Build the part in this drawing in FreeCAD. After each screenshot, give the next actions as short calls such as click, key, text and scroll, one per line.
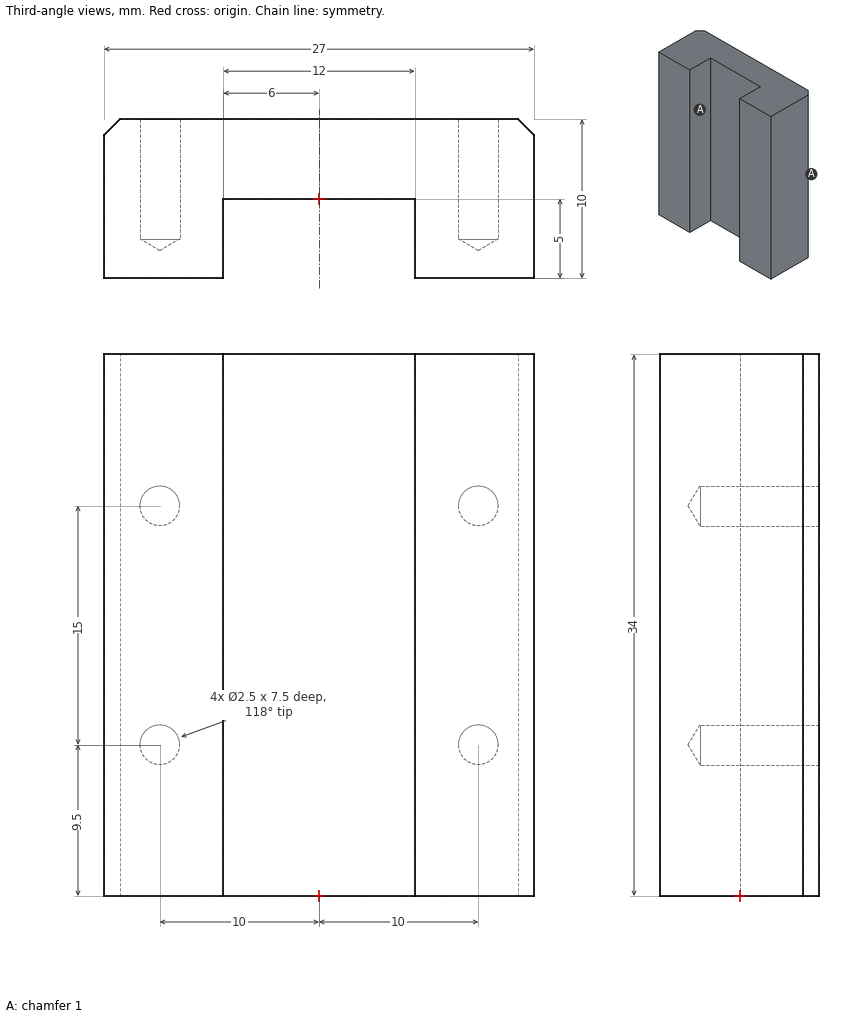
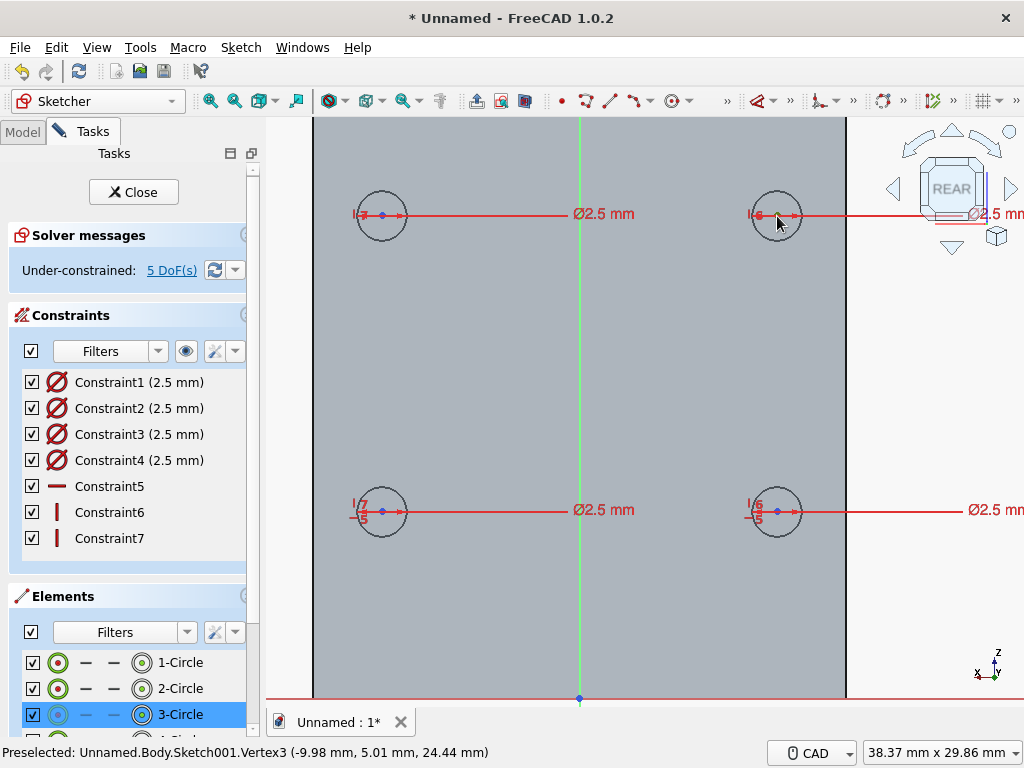
click(382, 216)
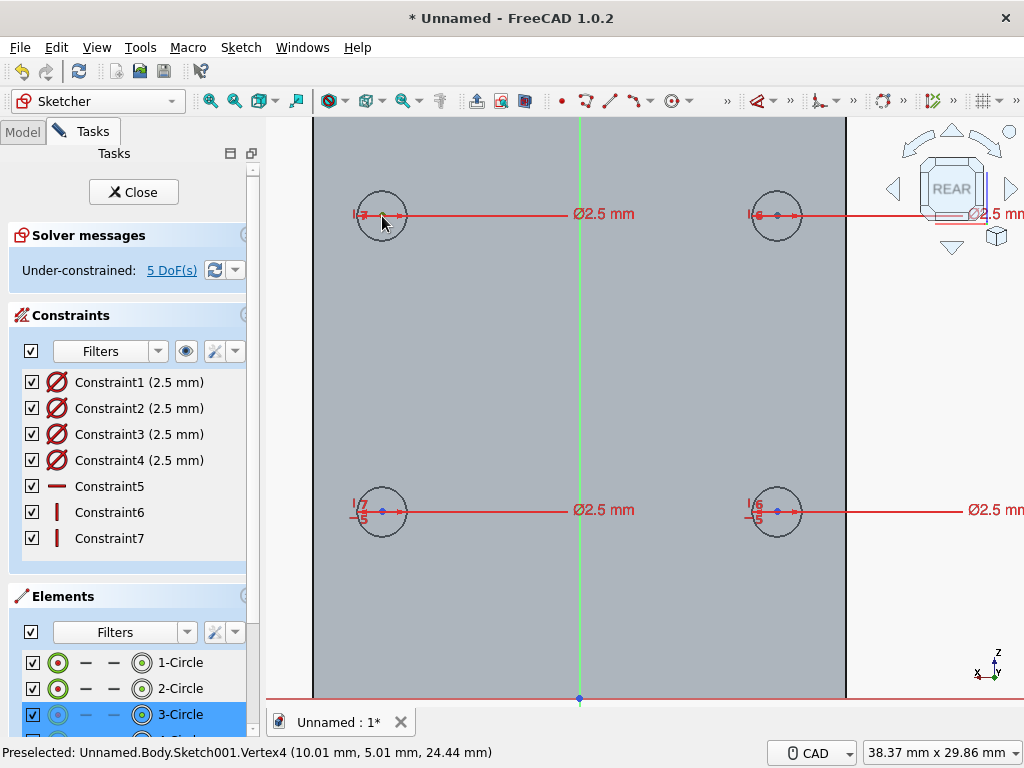
key(h)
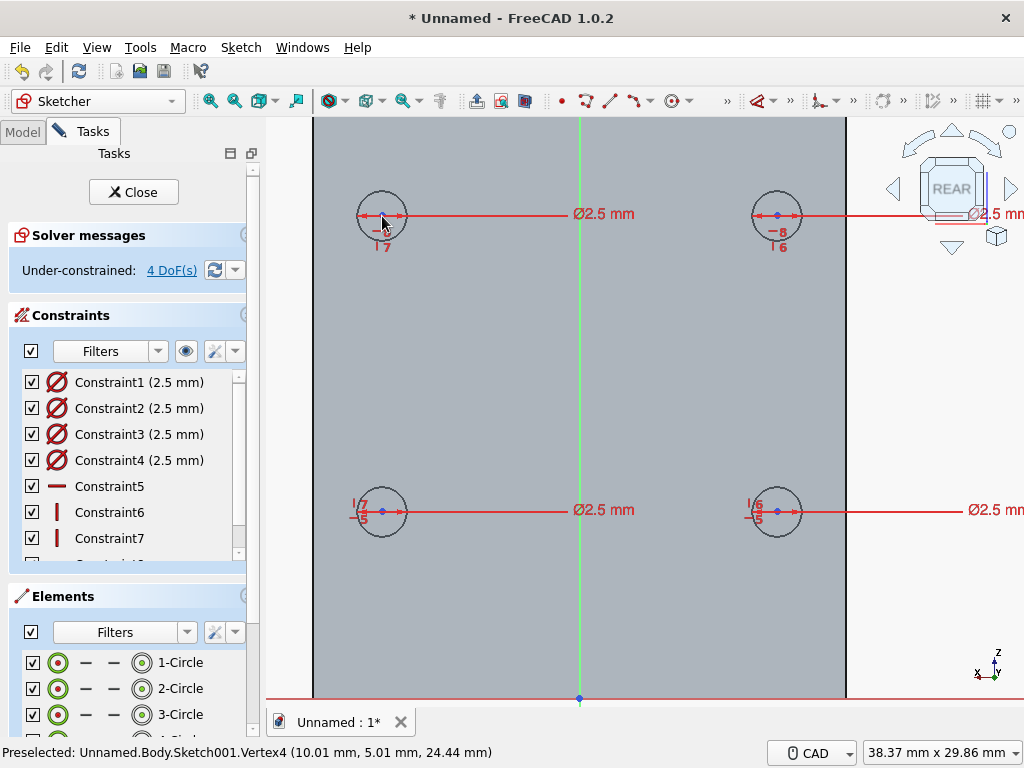
key(d)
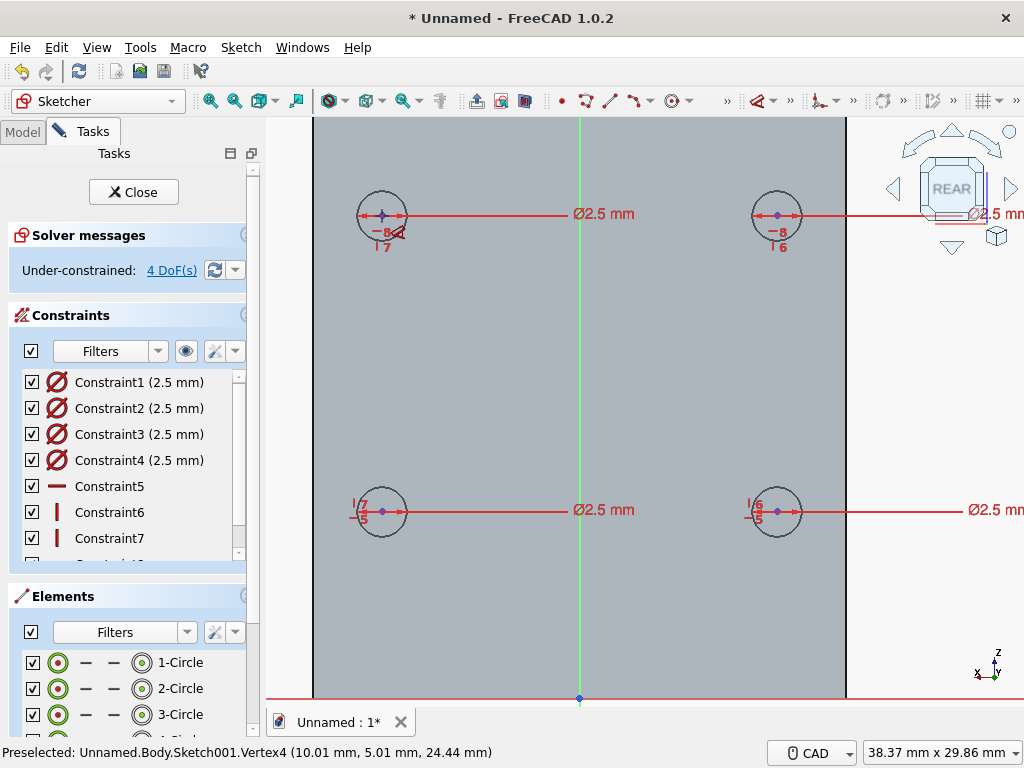
click(777, 512)
click(678, 478)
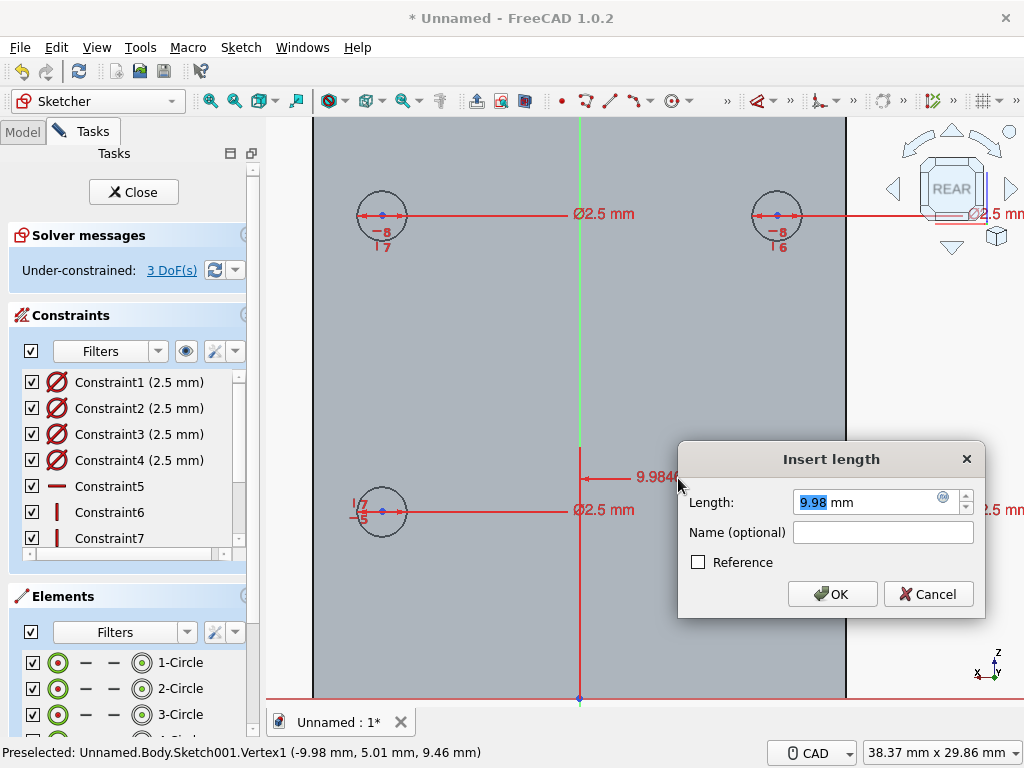
text(10)
key(Return)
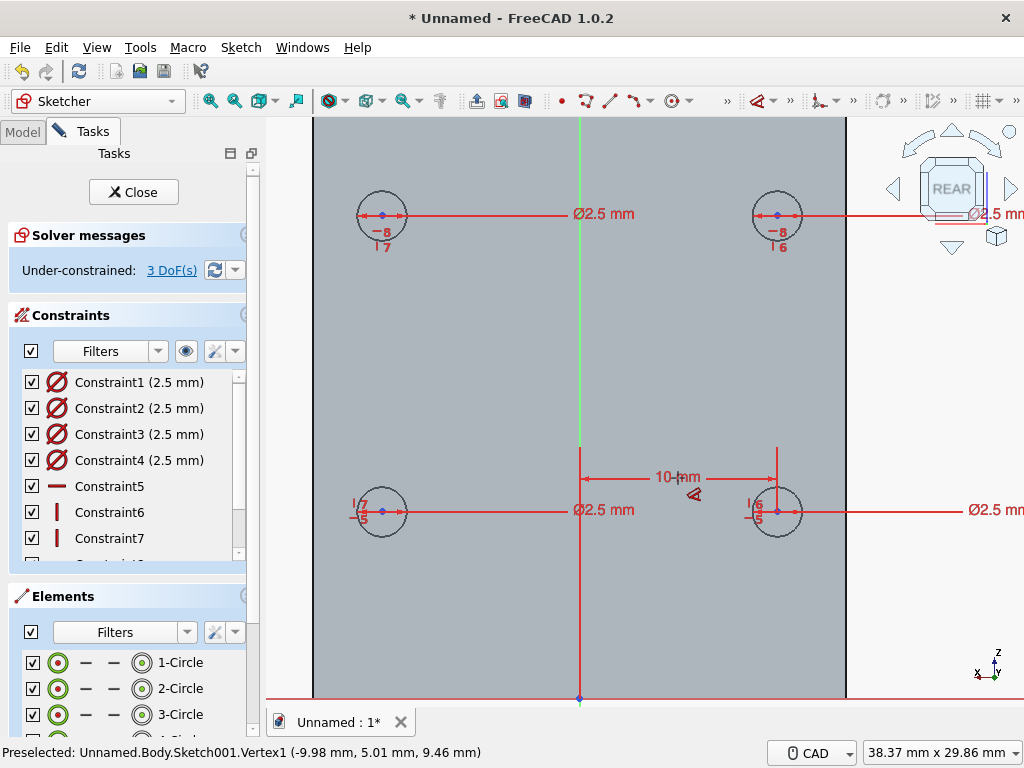
click(382, 512)
click(481, 478)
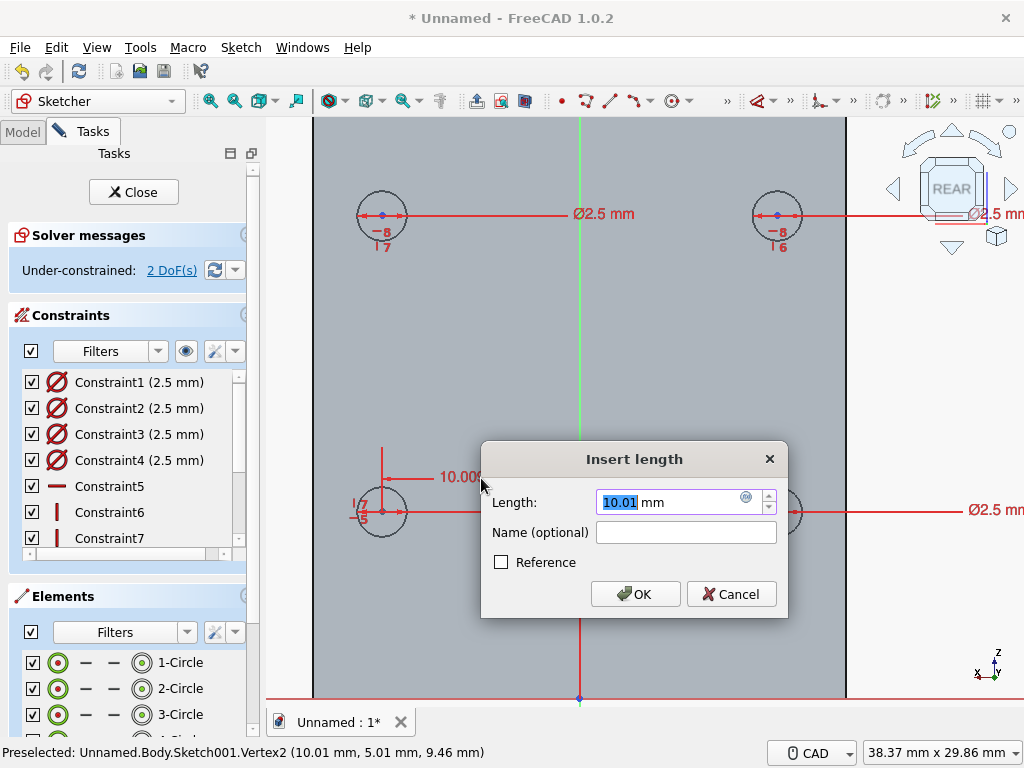
text(10)
key(Return)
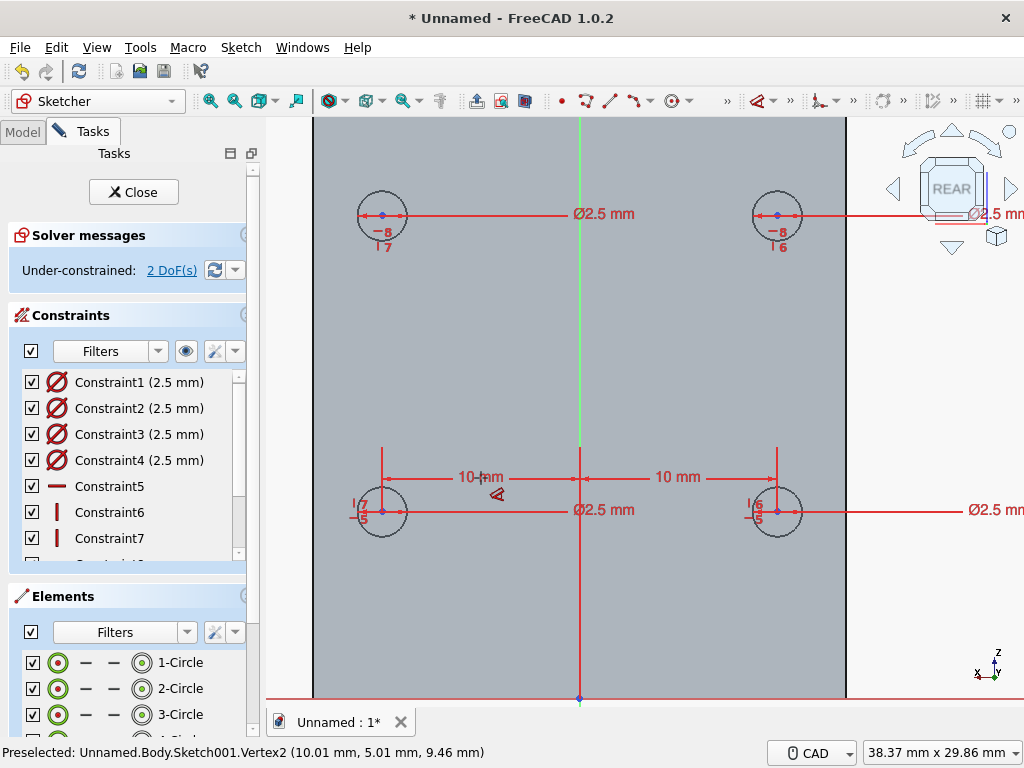
click(777, 512)
click(811, 596)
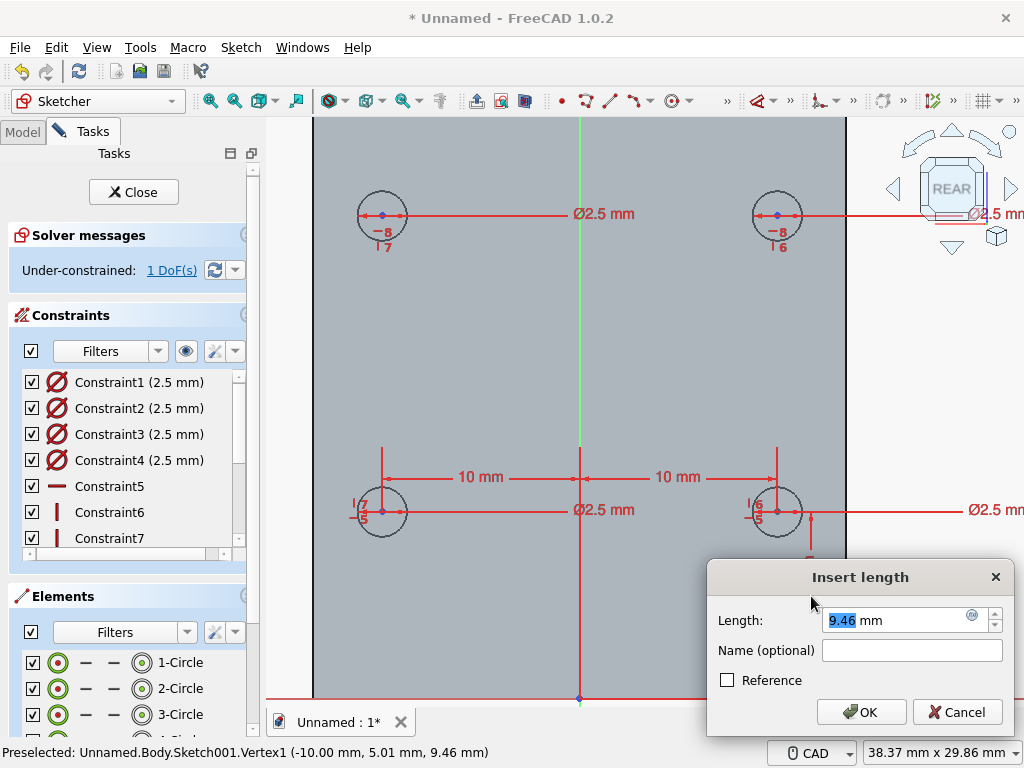
text(9.5)
key(Return)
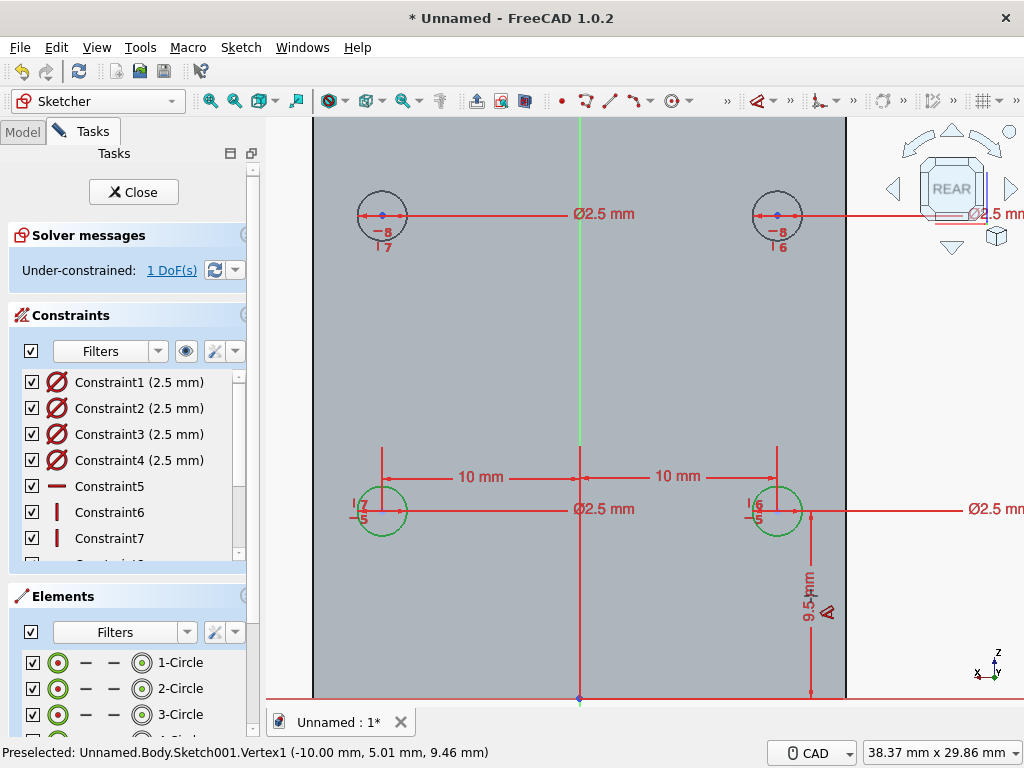
click(777, 511)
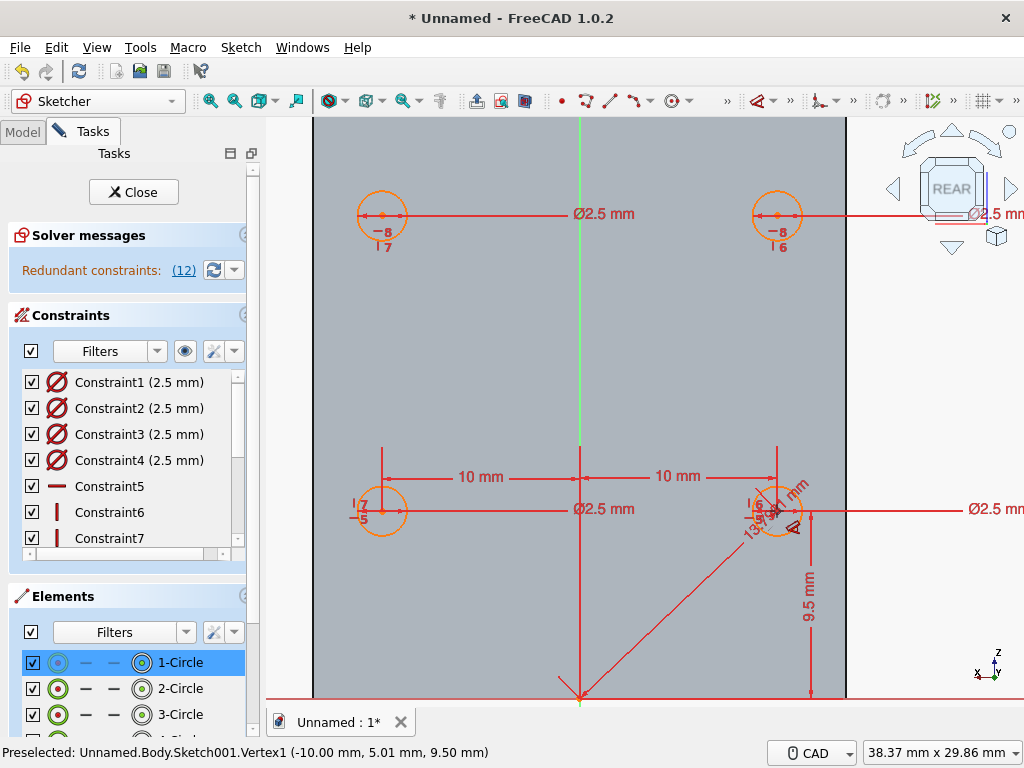
click(777, 216)
click(811, 364)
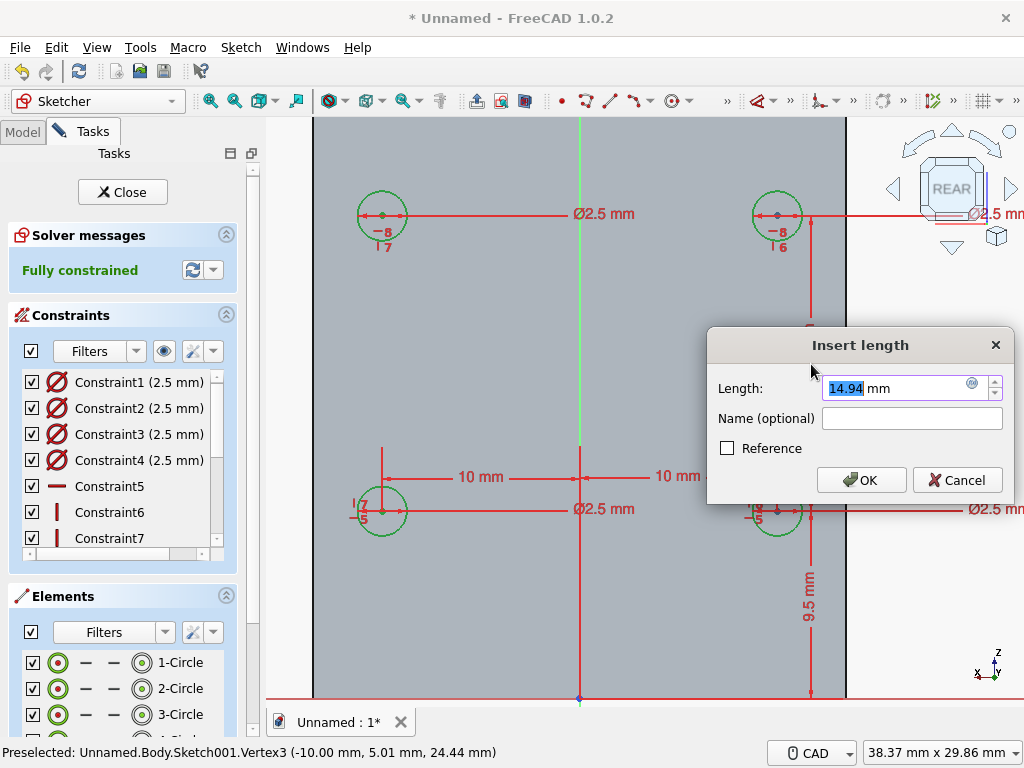
text(15)
key(Return)
key(Escape)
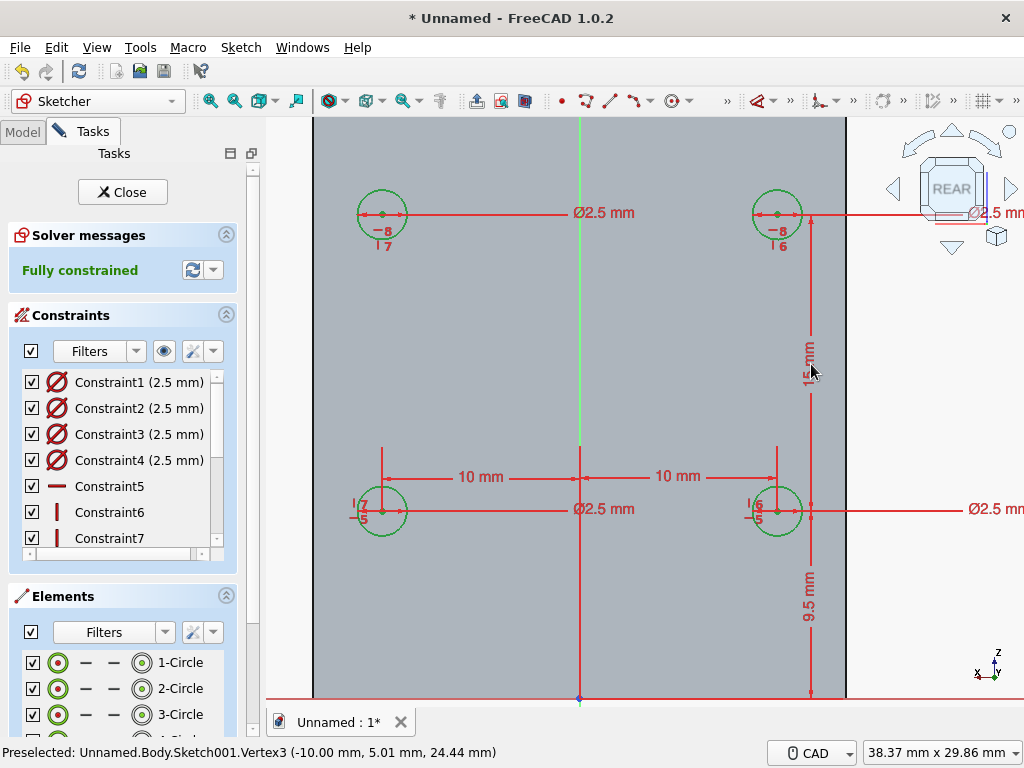
click(123, 192)